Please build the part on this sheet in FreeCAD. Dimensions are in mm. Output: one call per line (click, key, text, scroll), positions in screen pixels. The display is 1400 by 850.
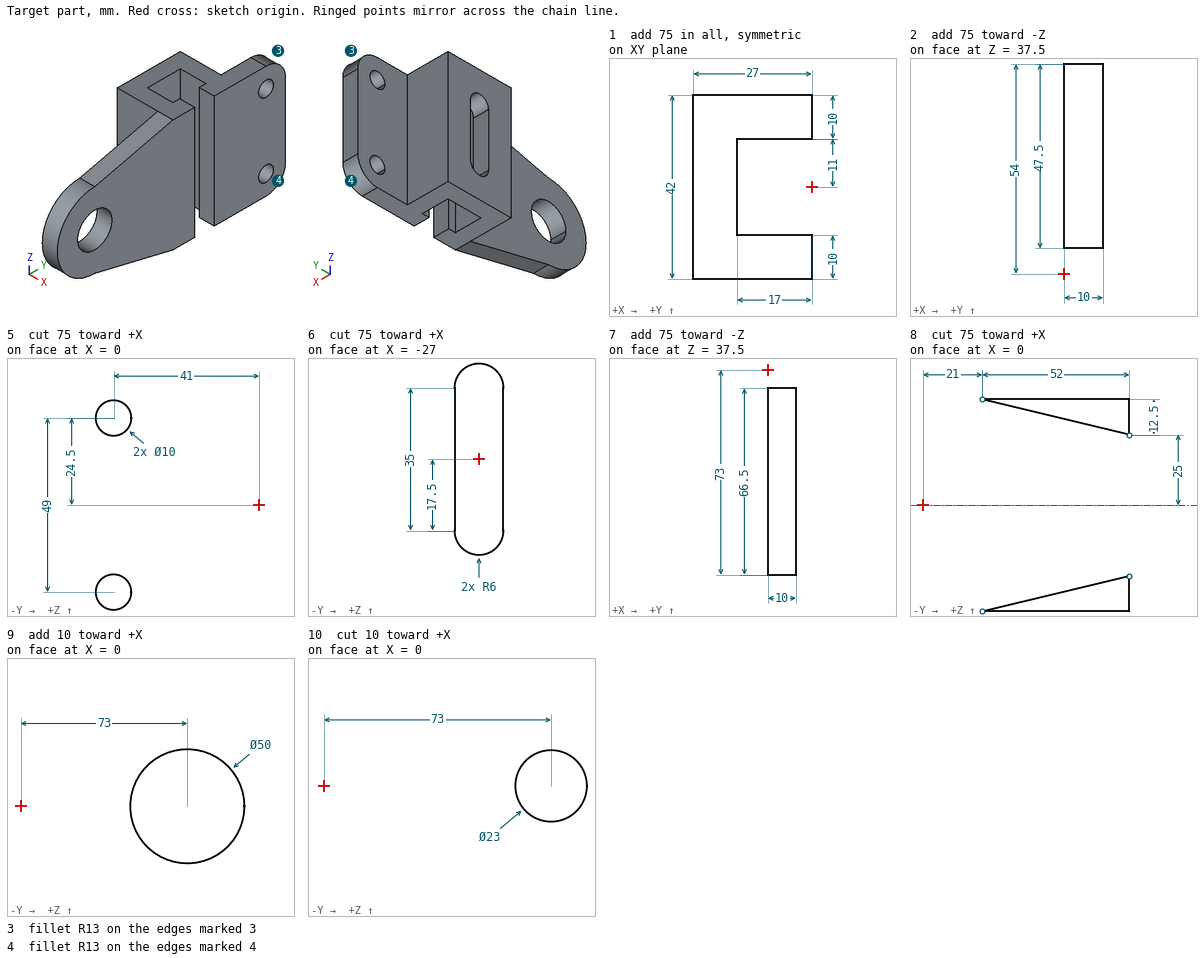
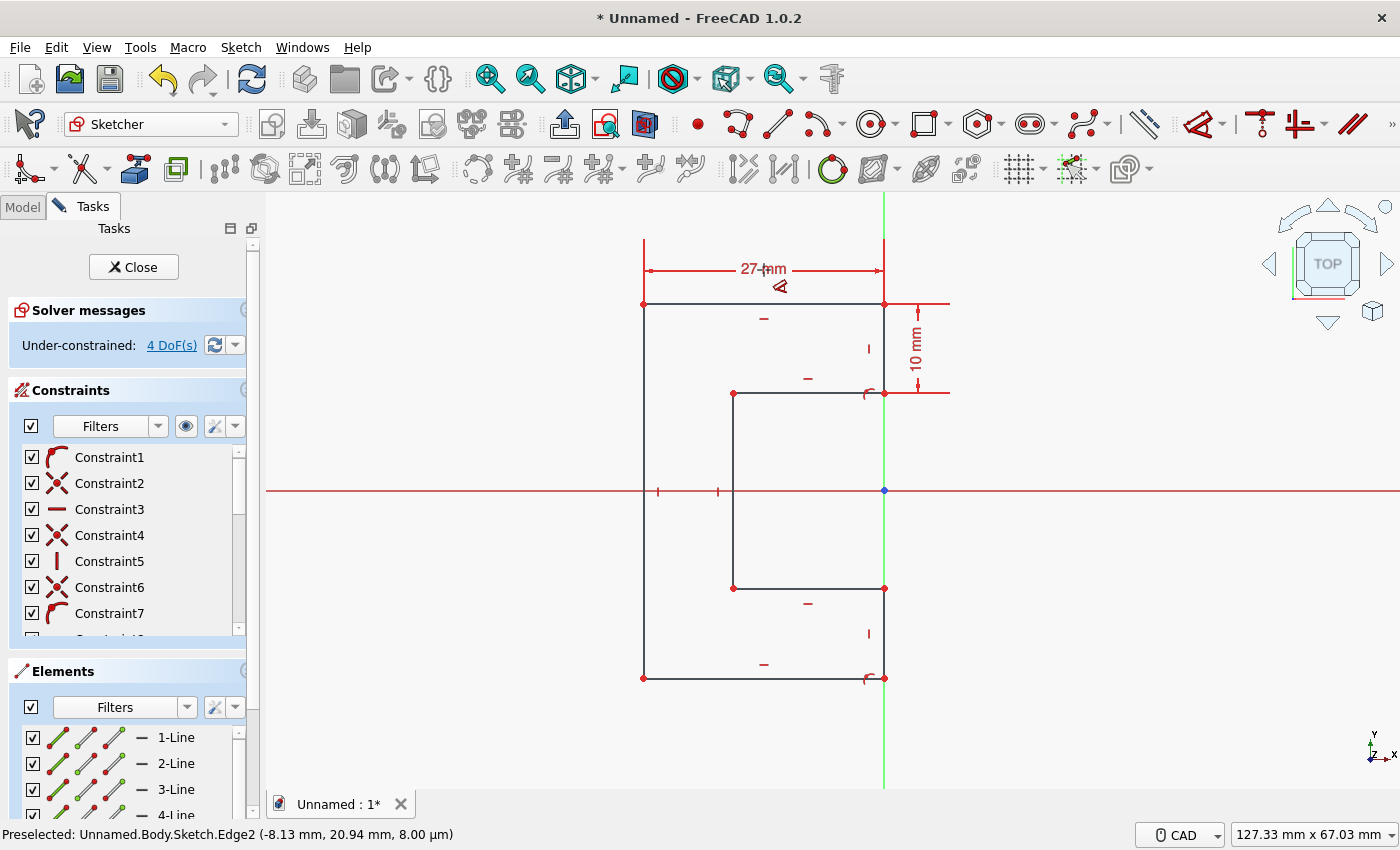
click(644, 417)
click(610, 405)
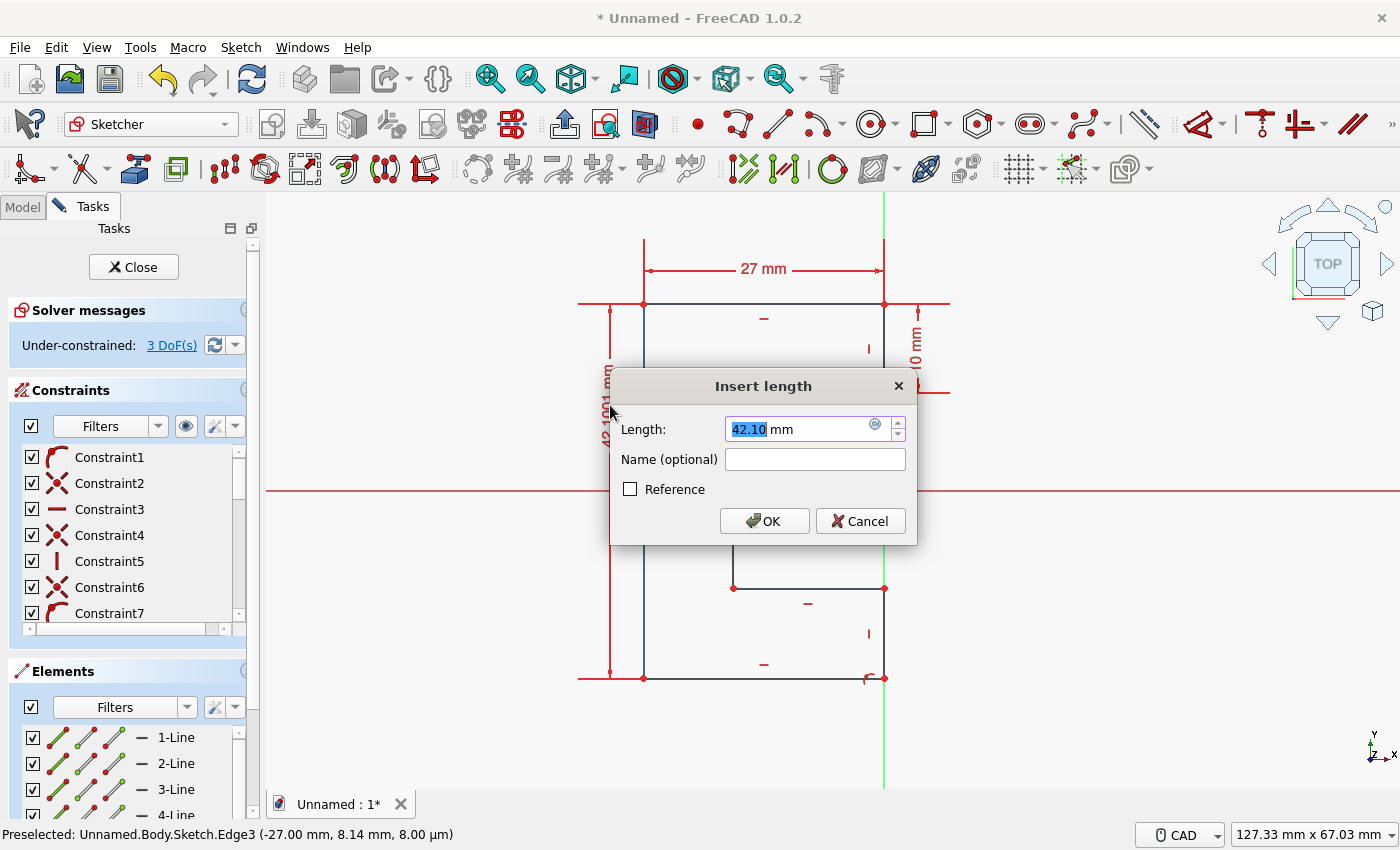
text(42)
key(Return)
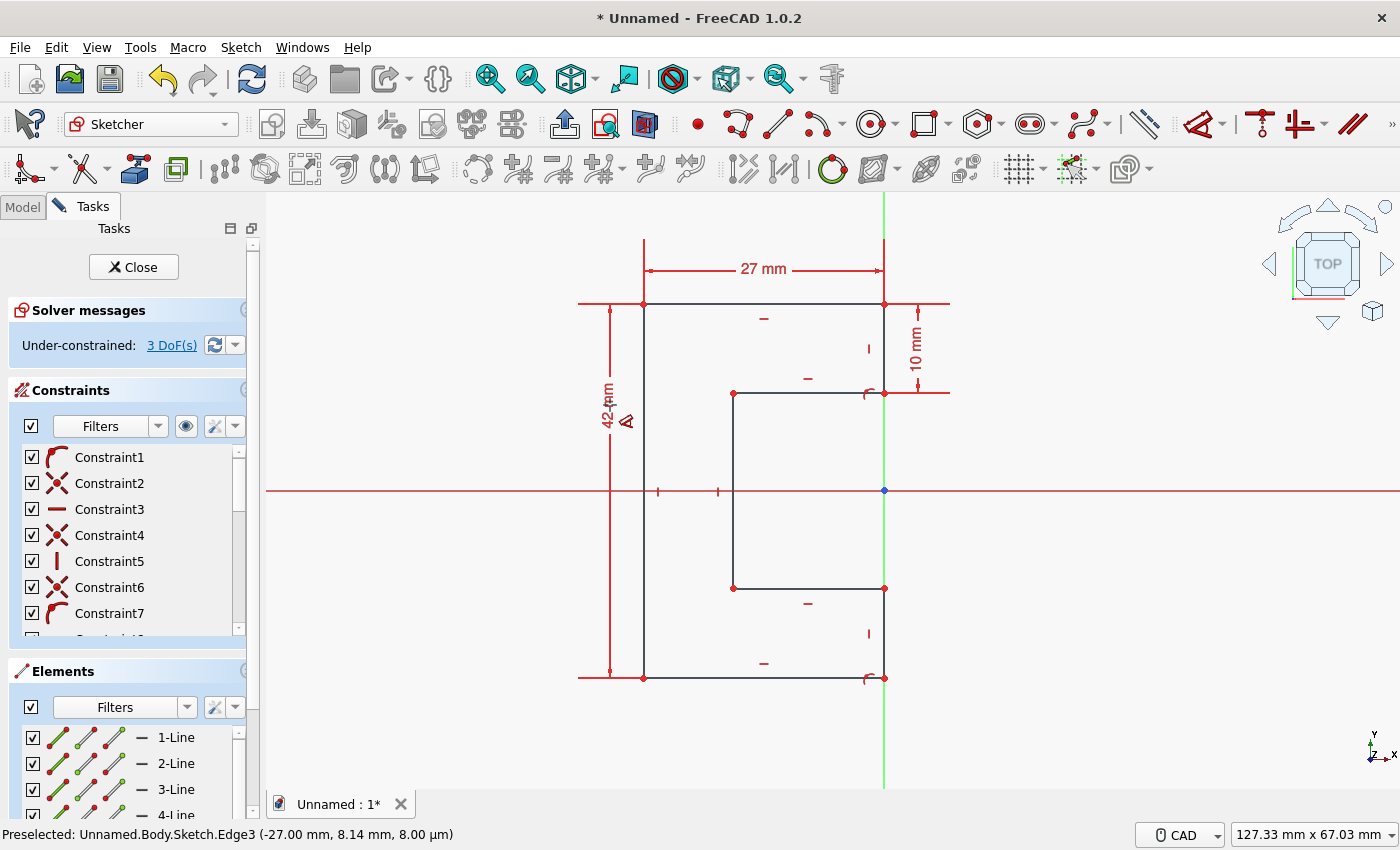
click(884, 651)
click(918, 634)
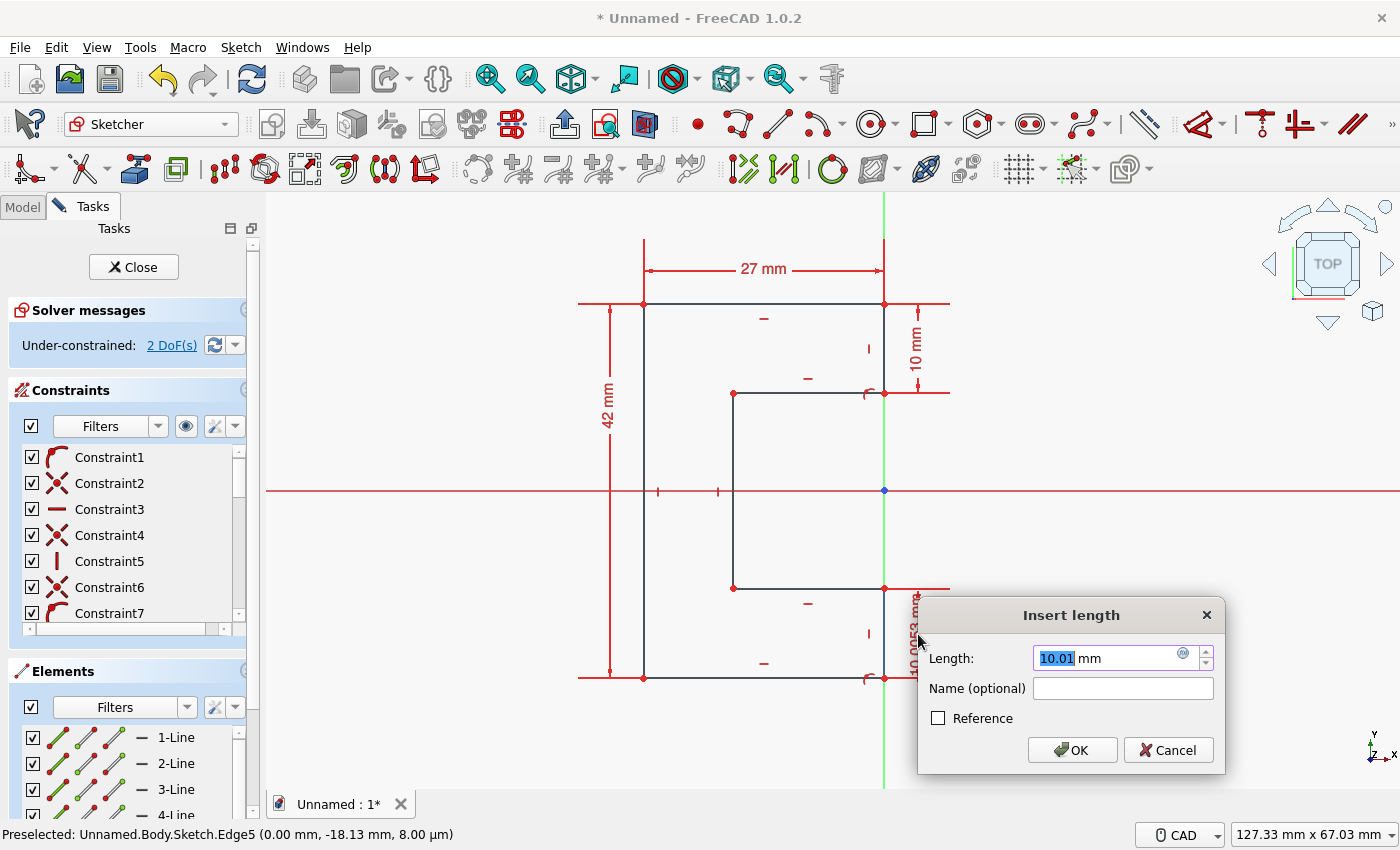
text(10)
key(Return)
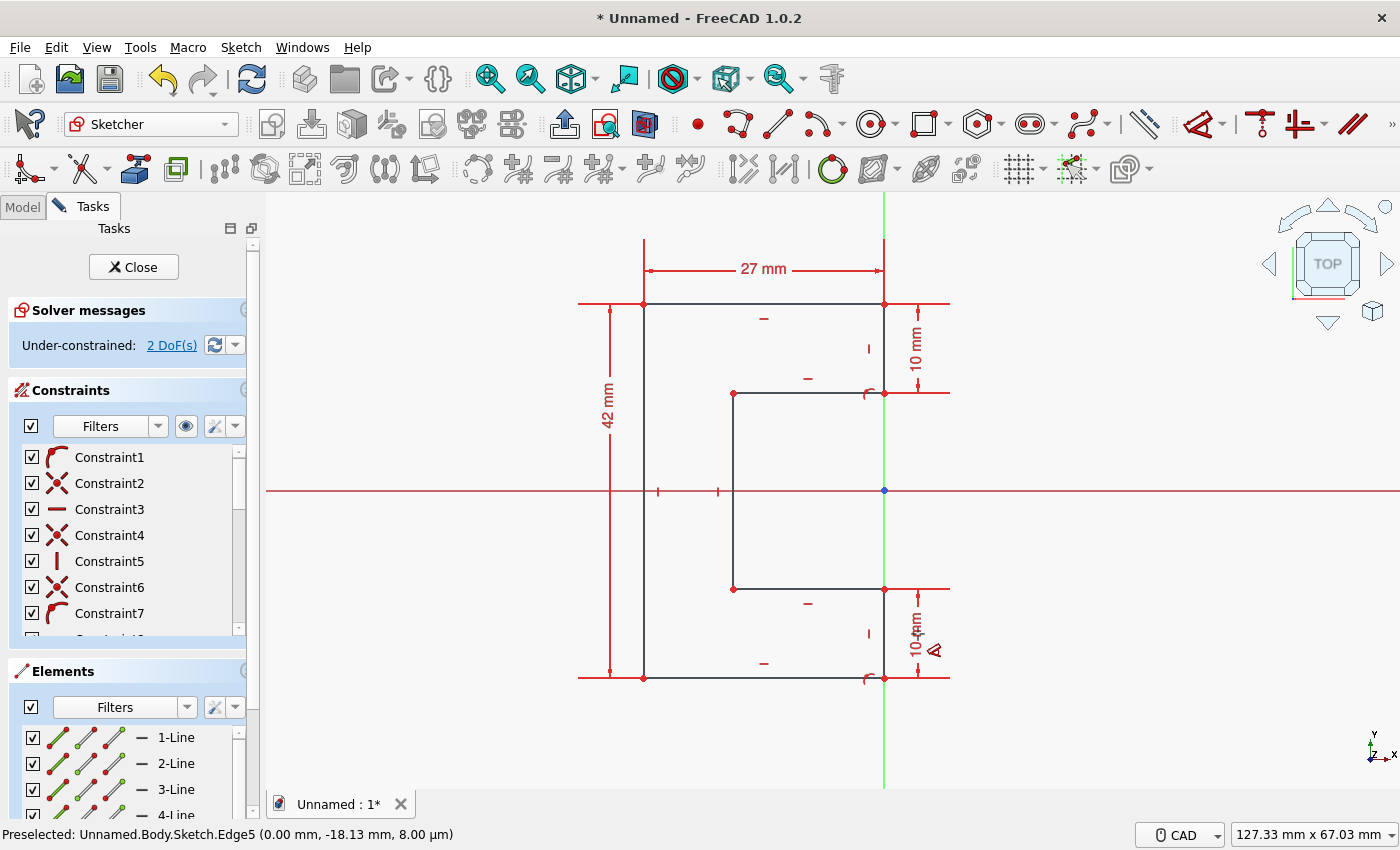
click(839, 589)
click(809, 623)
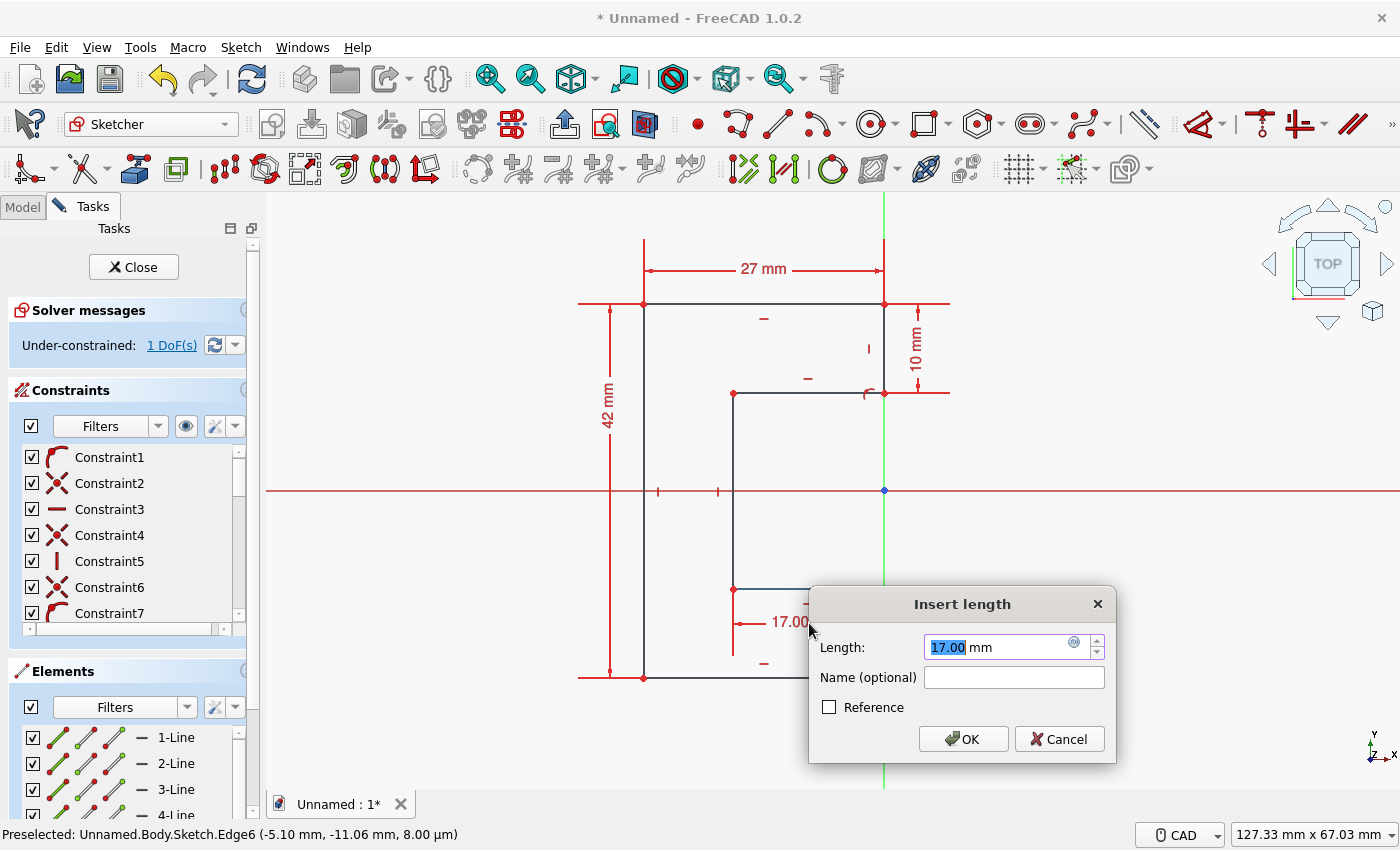
text(17)
key(Return)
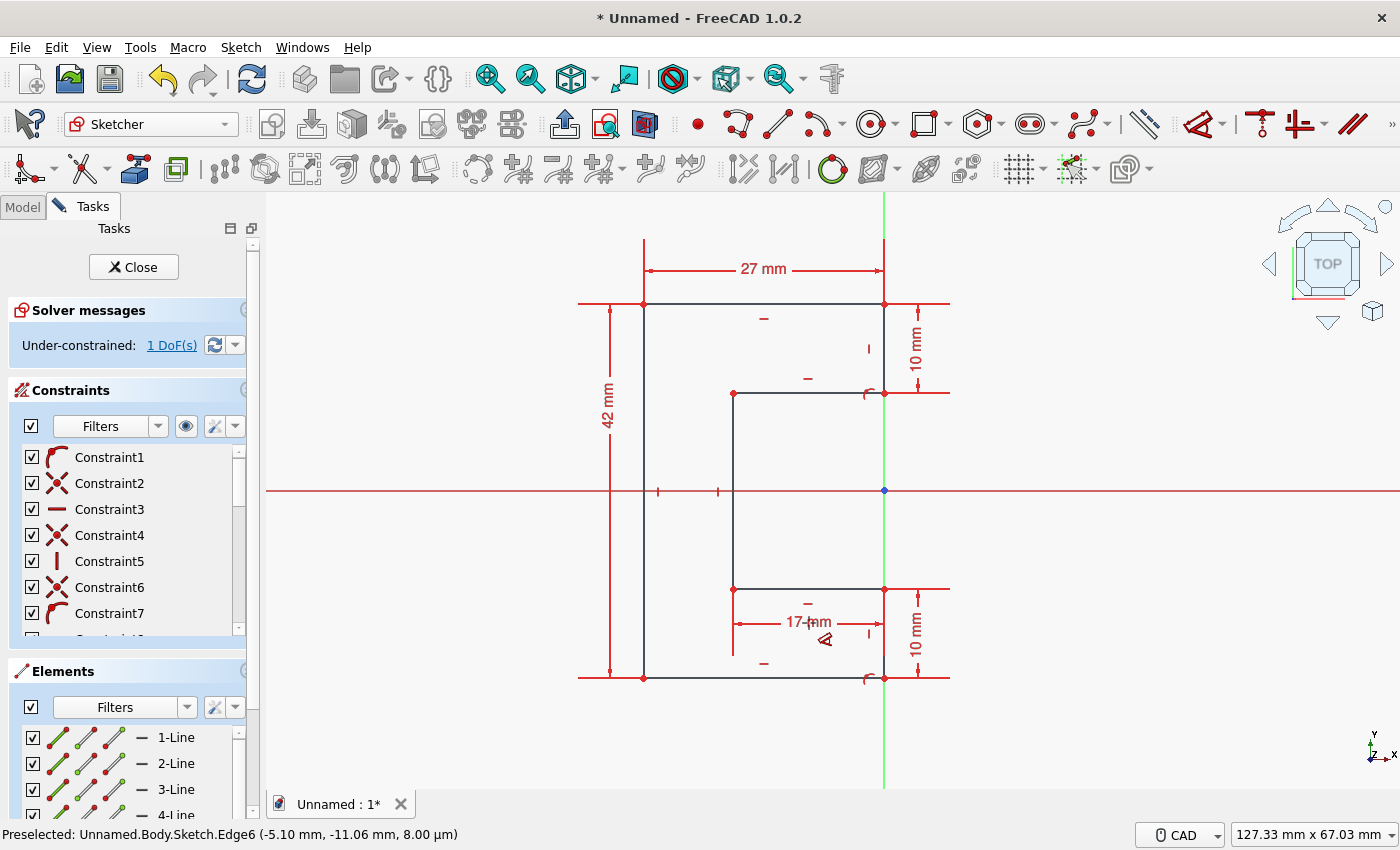
click(884, 393)
click(918, 442)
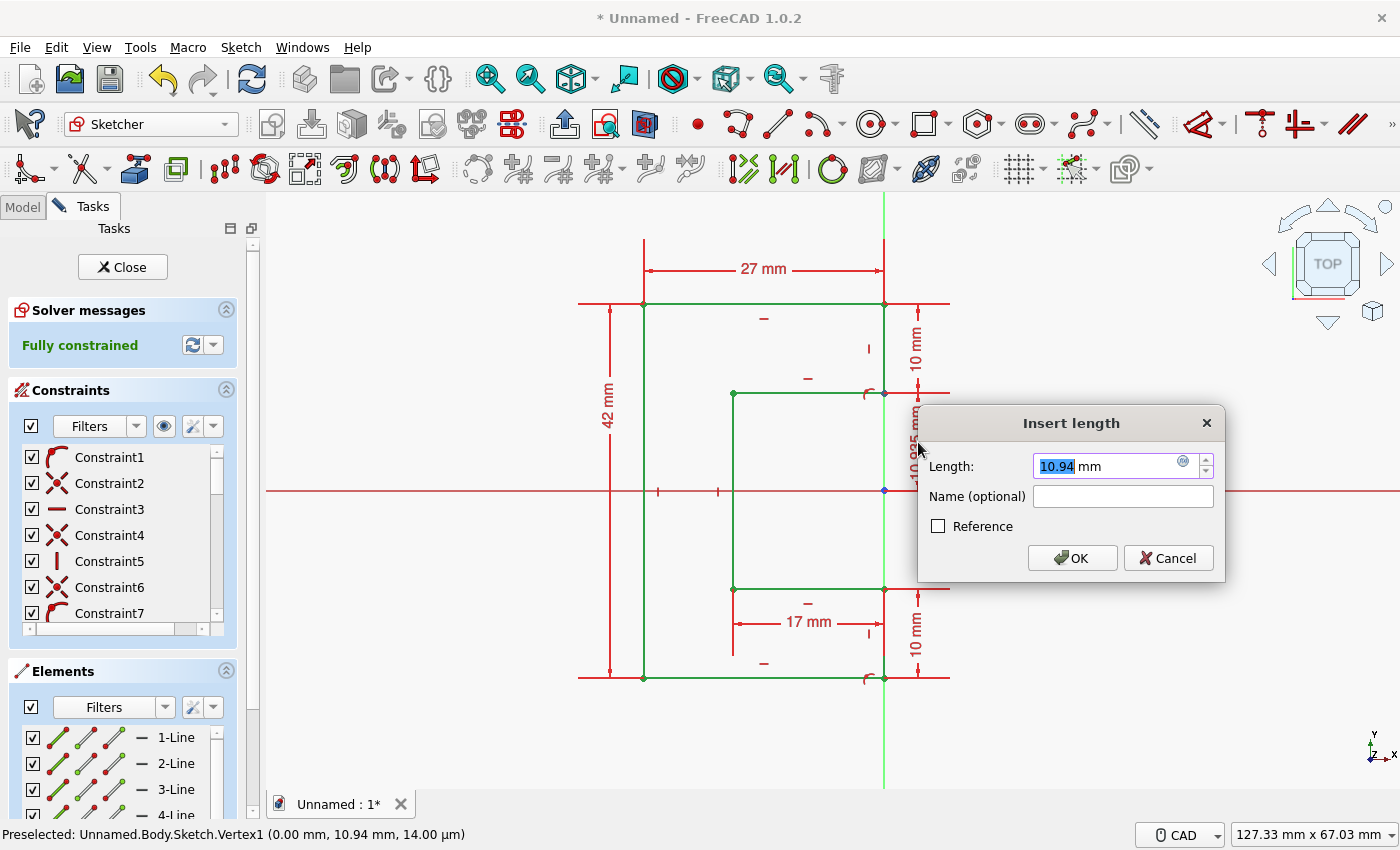
text(11)
key(Return)
key(Escape)